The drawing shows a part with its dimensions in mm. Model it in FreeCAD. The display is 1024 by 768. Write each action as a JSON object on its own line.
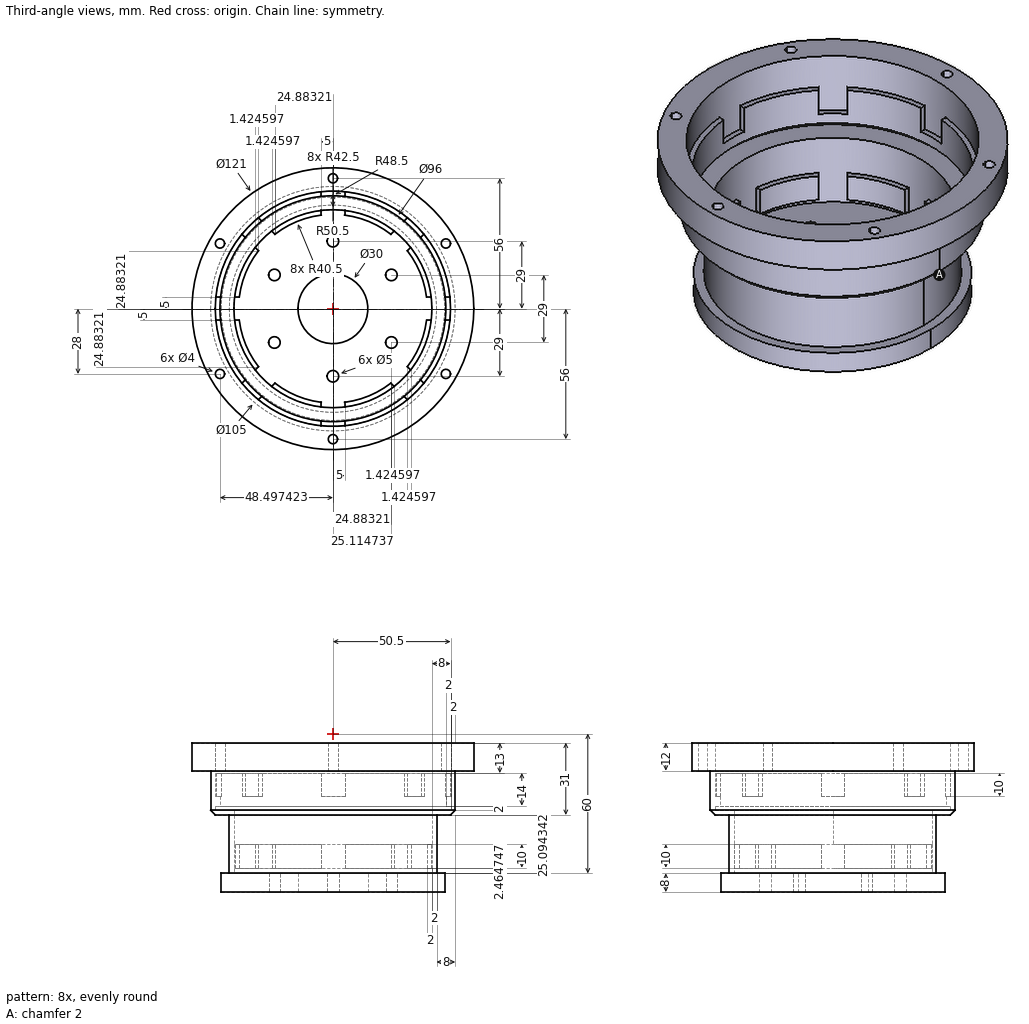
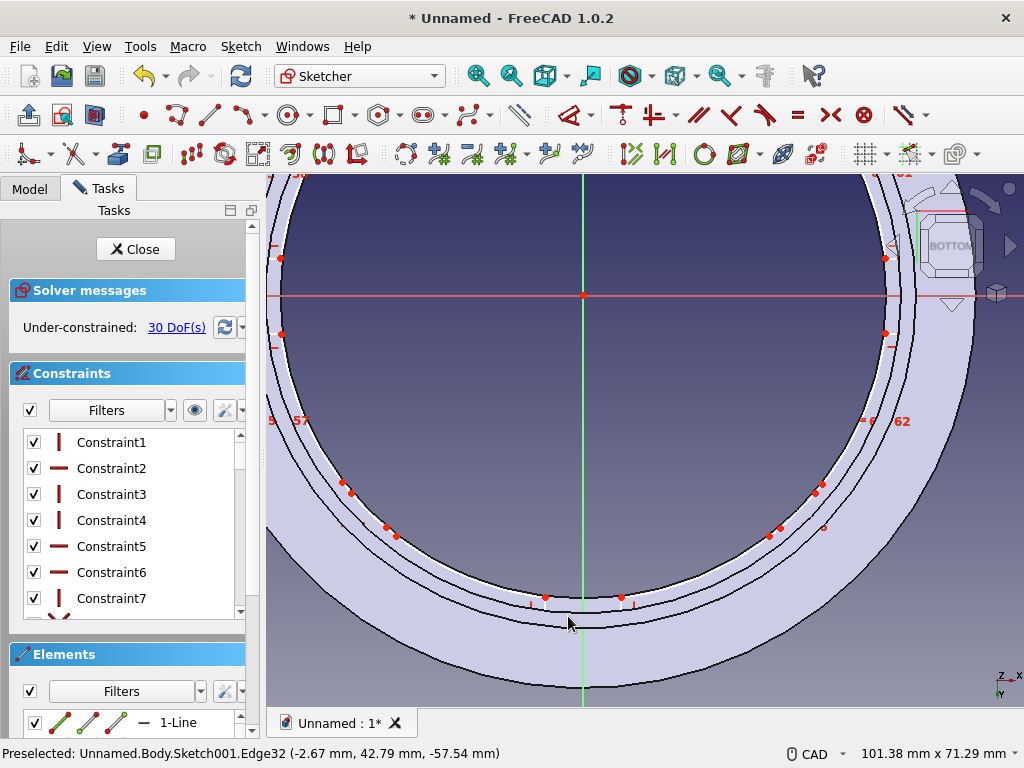
{"action": "key", "text": "e"}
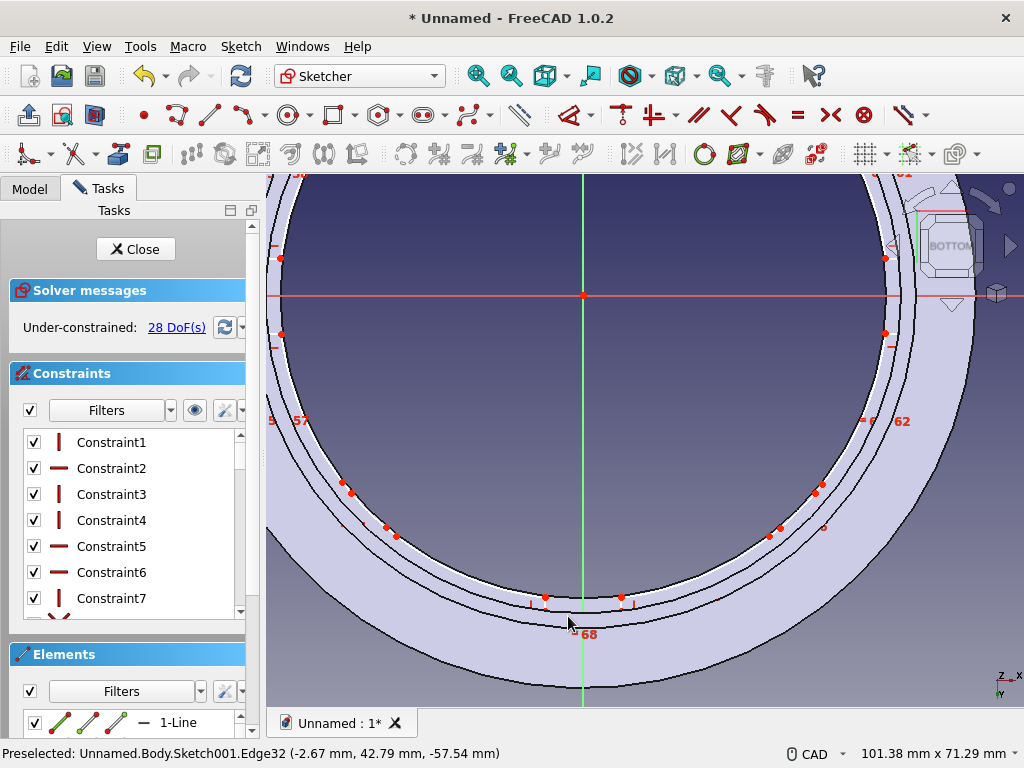
{"action": "scroll", "coordinate": [568, 617], "scroll_direction": "down", "scroll_amount": 3}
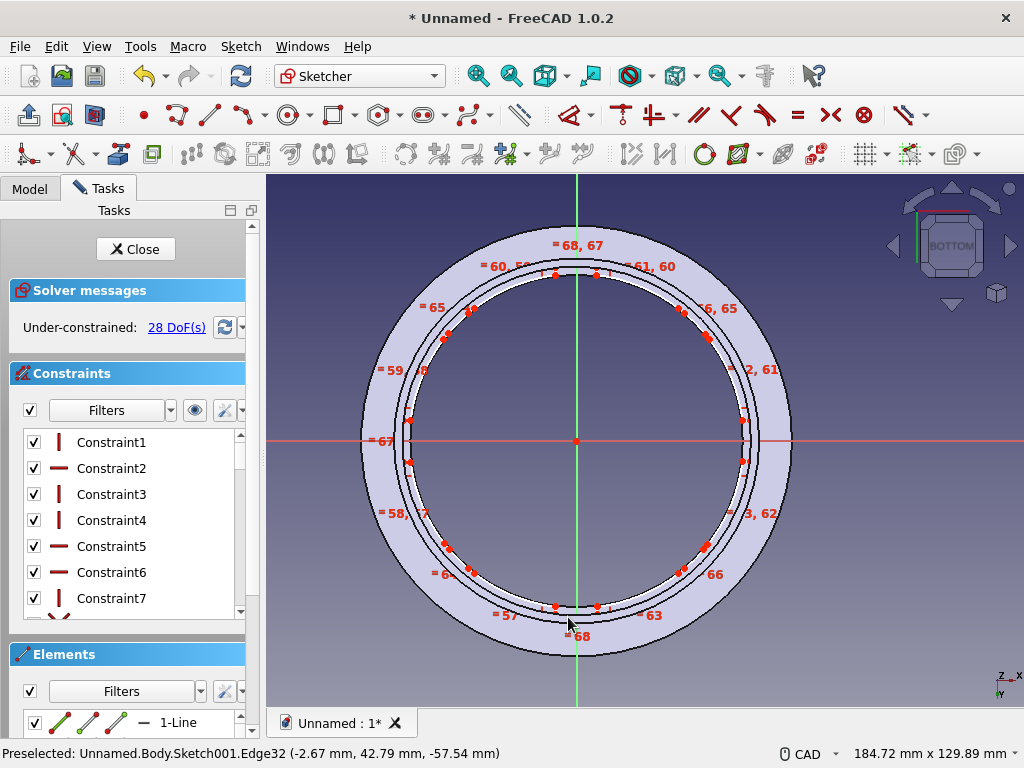
{"action": "scroll", "coordinate": [403, 421], "scroll_direction": "up", "scroll_amount": 3}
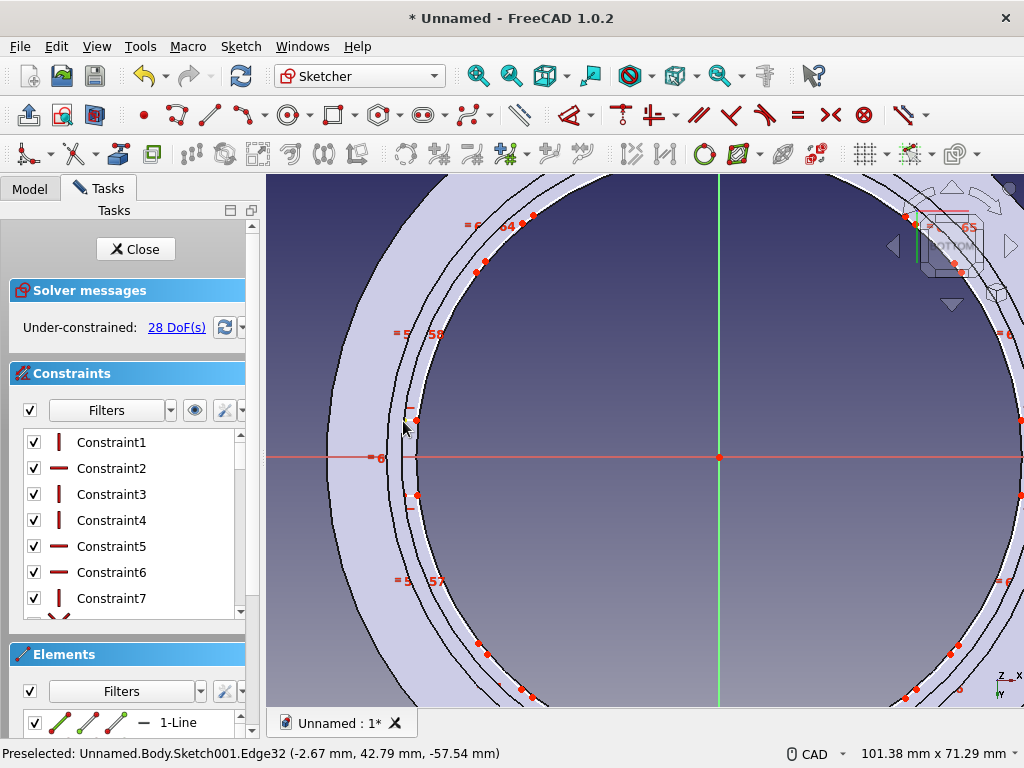
{"action": "left_click", "coordinate": [403, 420]}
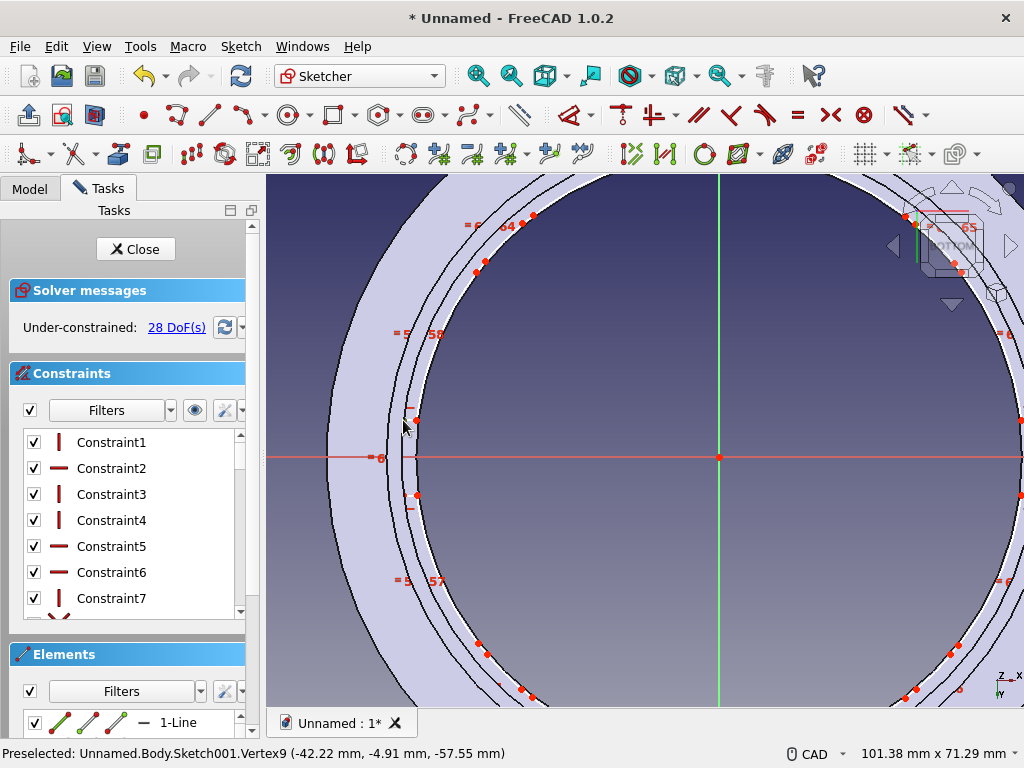
{"action": "scroll", "coordinate": [403, 420], "scroll_direction": "down", "scroll_amount": 3}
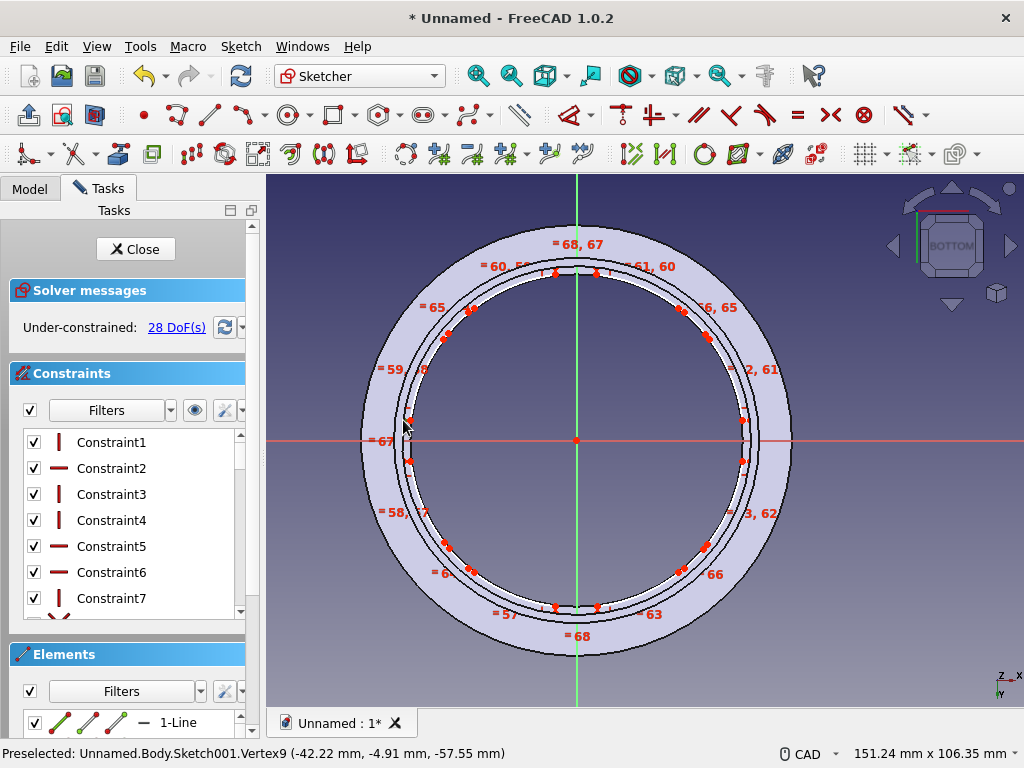
{"action": "scroll", "coordinate": [751, 420], "scroll_direction": "up", "scroll_amount": 2}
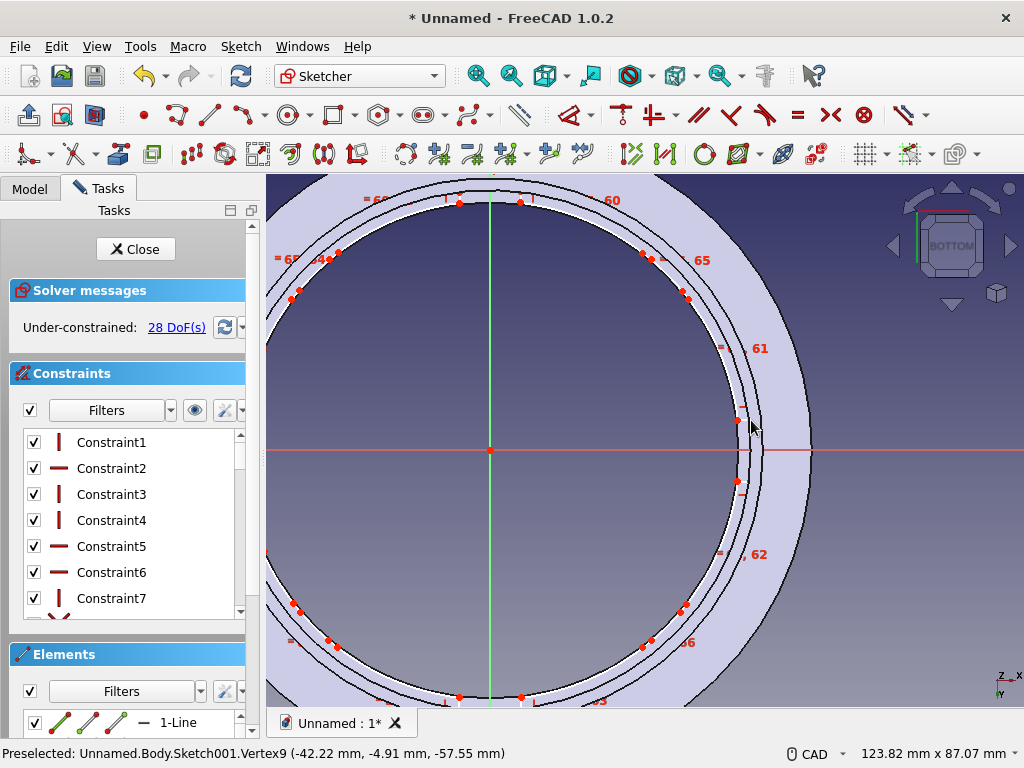
{"action": "left_click", "coordinate": [750, 420]}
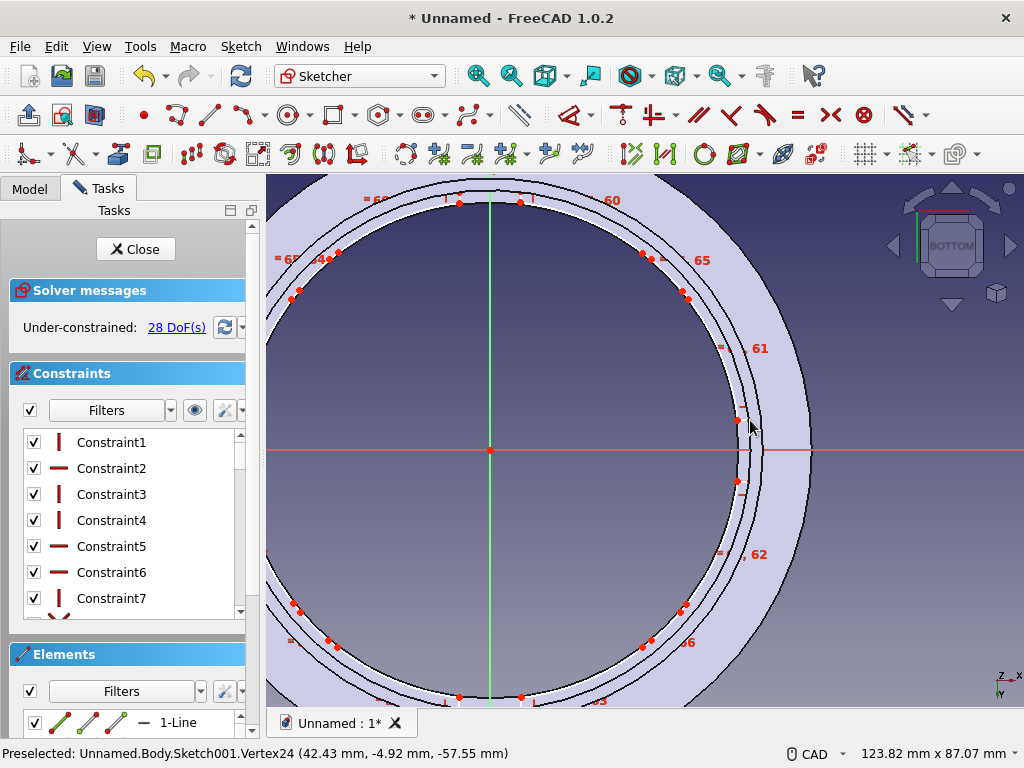
{"action": "left_click", "coordinate": [490, 645]}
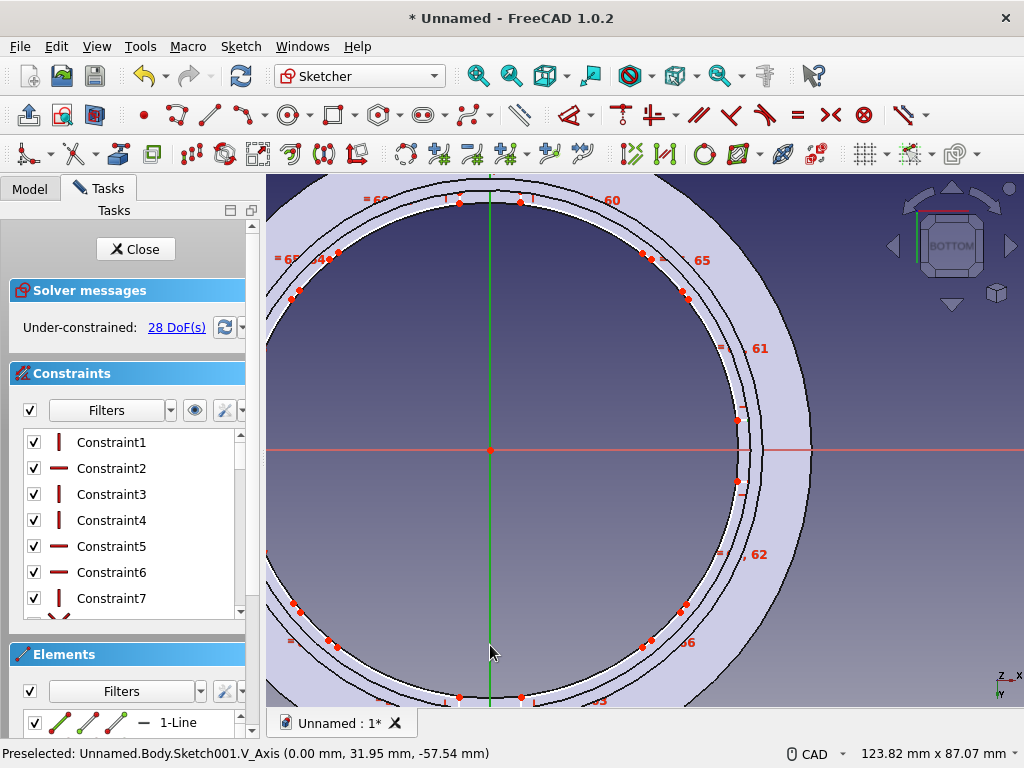
{"action": "key", "text": "s"}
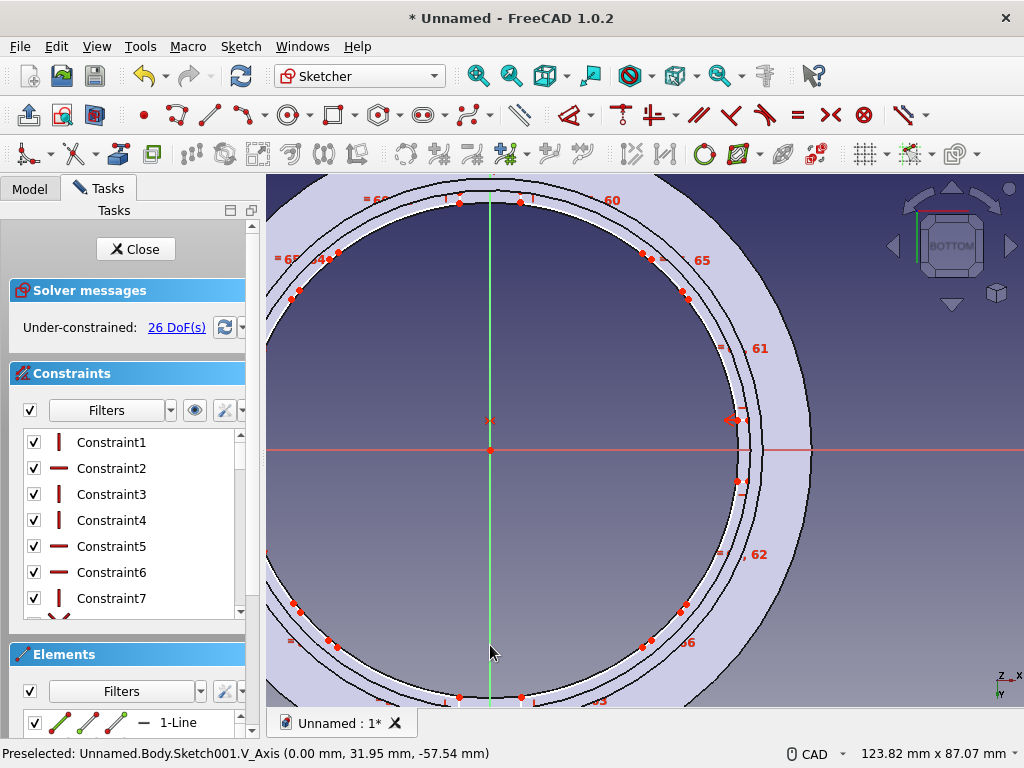
{"action": "key", "text": "d"}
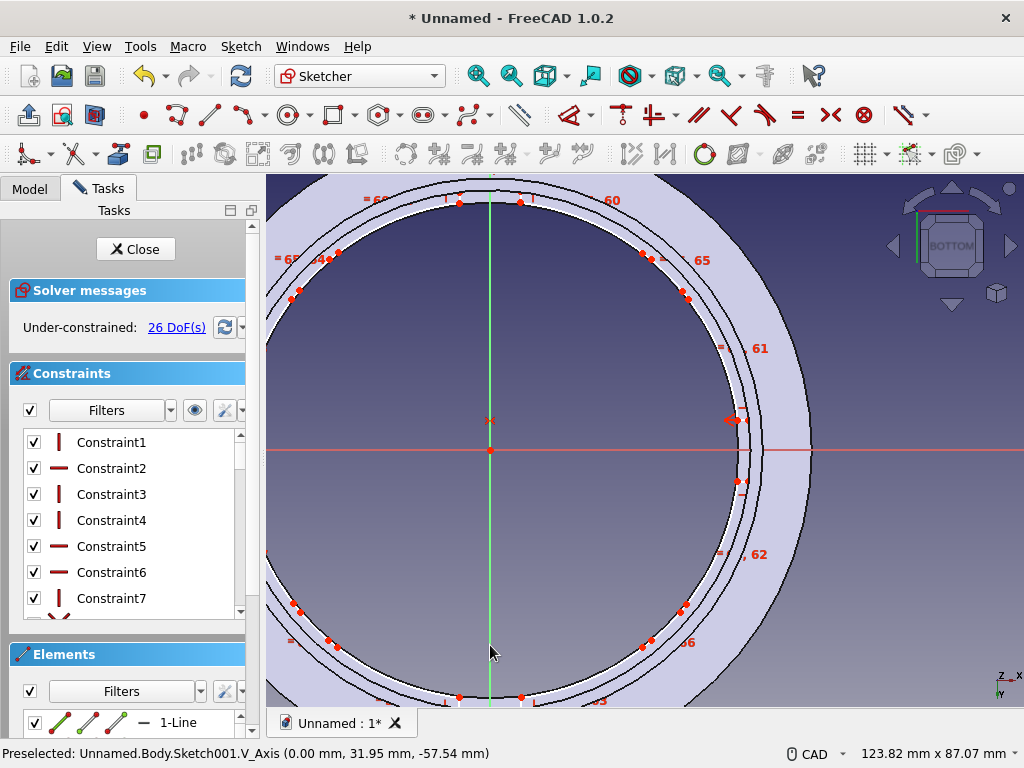
{"action": "left_click", "coordinate": [371, 669]}
{"action": "left_click", "coordinate": [737, 585]}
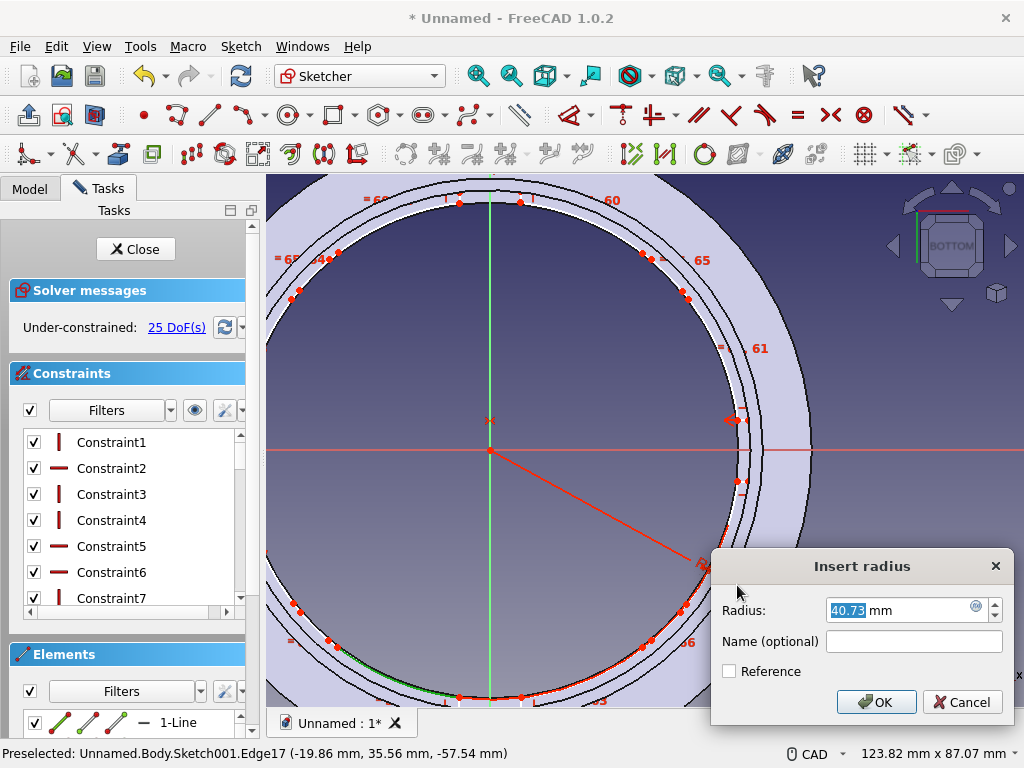
{"action": "type", "text": "40.5"}
{"action": "key", "text": "Return"}